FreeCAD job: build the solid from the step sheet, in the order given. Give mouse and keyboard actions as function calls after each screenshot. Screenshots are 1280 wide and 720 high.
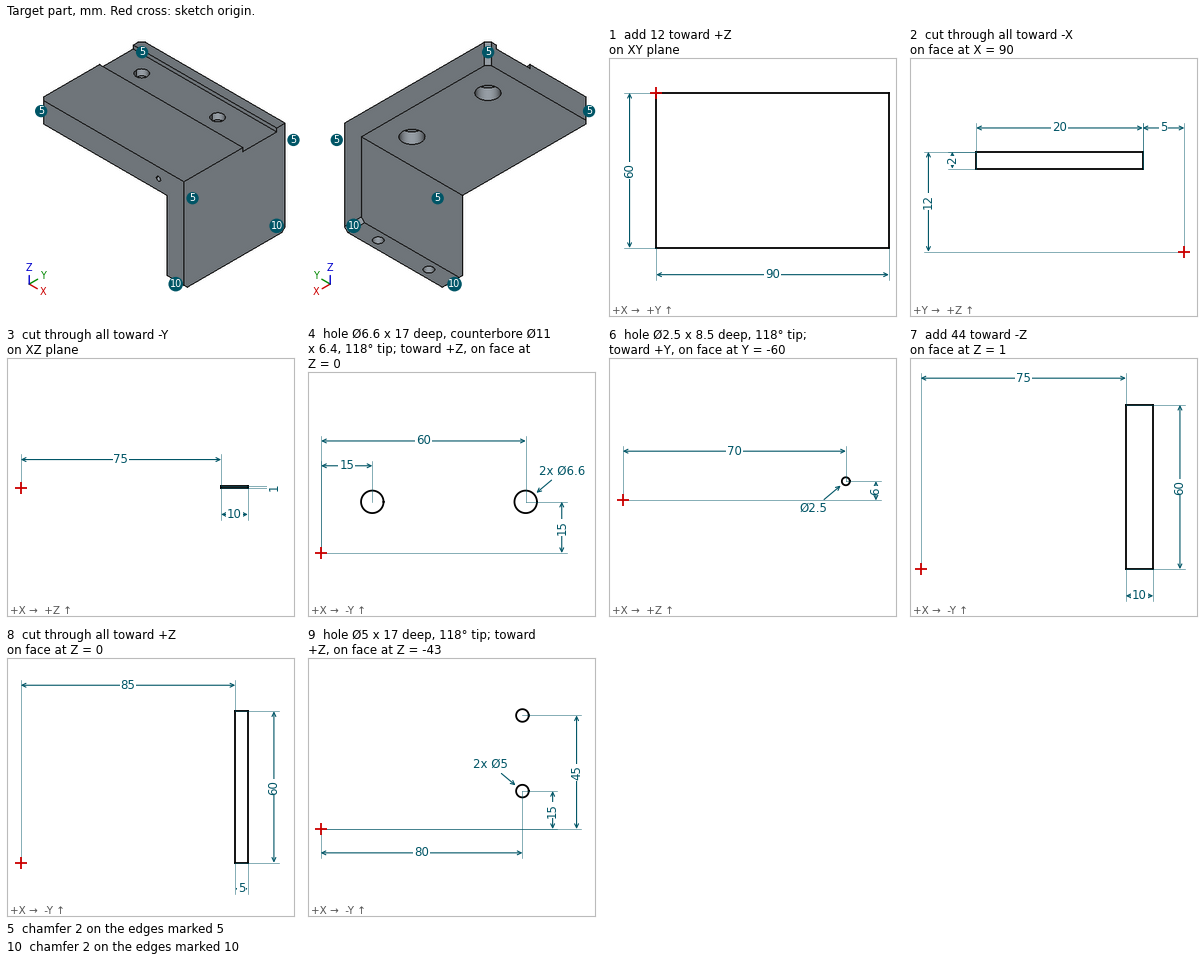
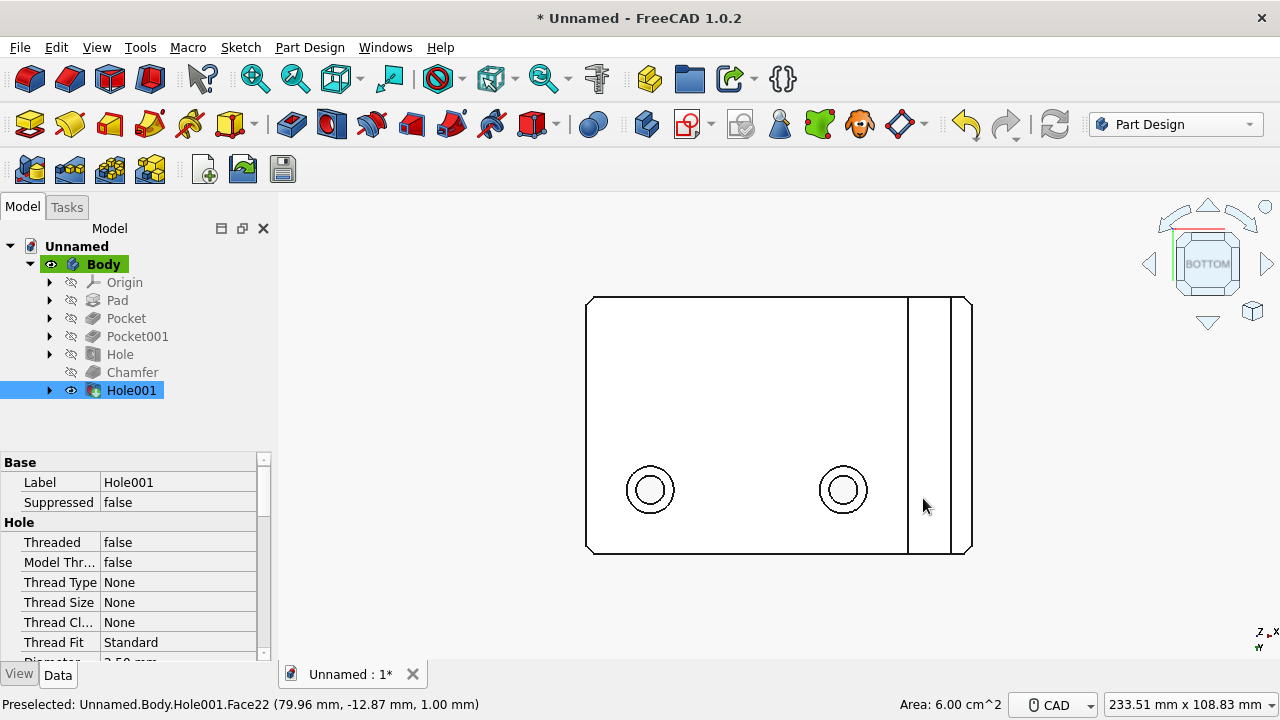
click(688, 124)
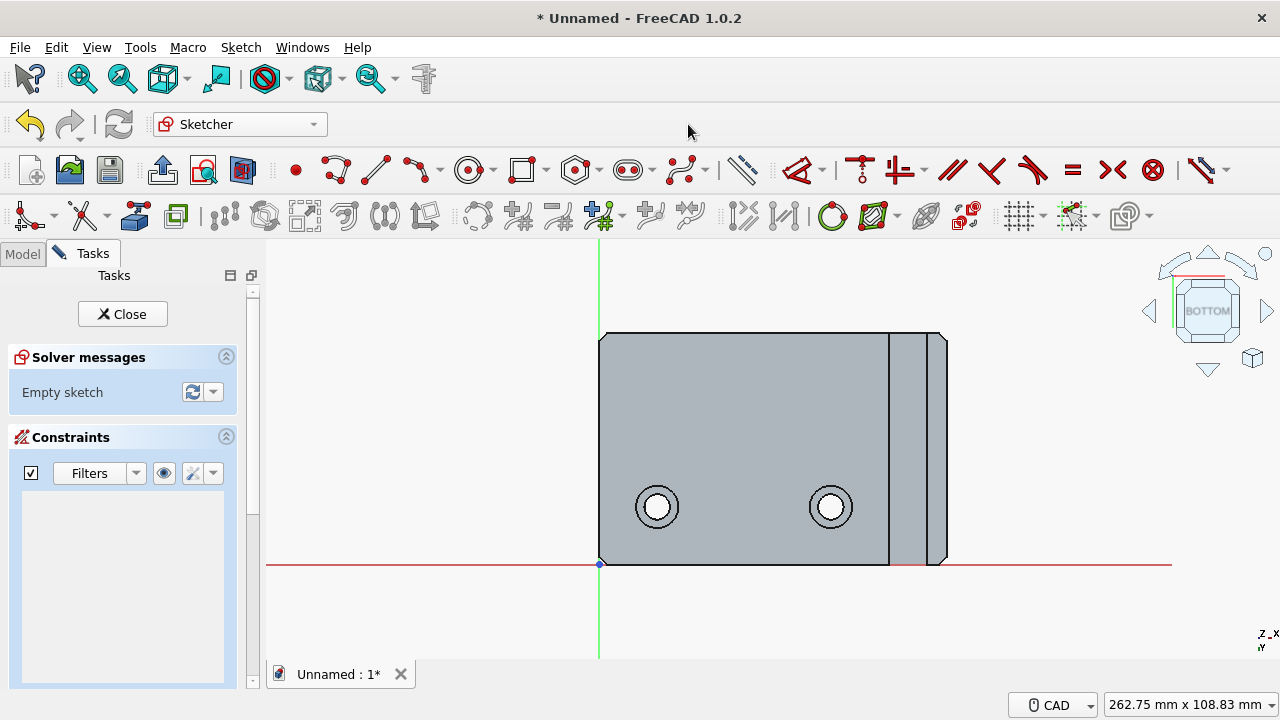
key(q)
key(s)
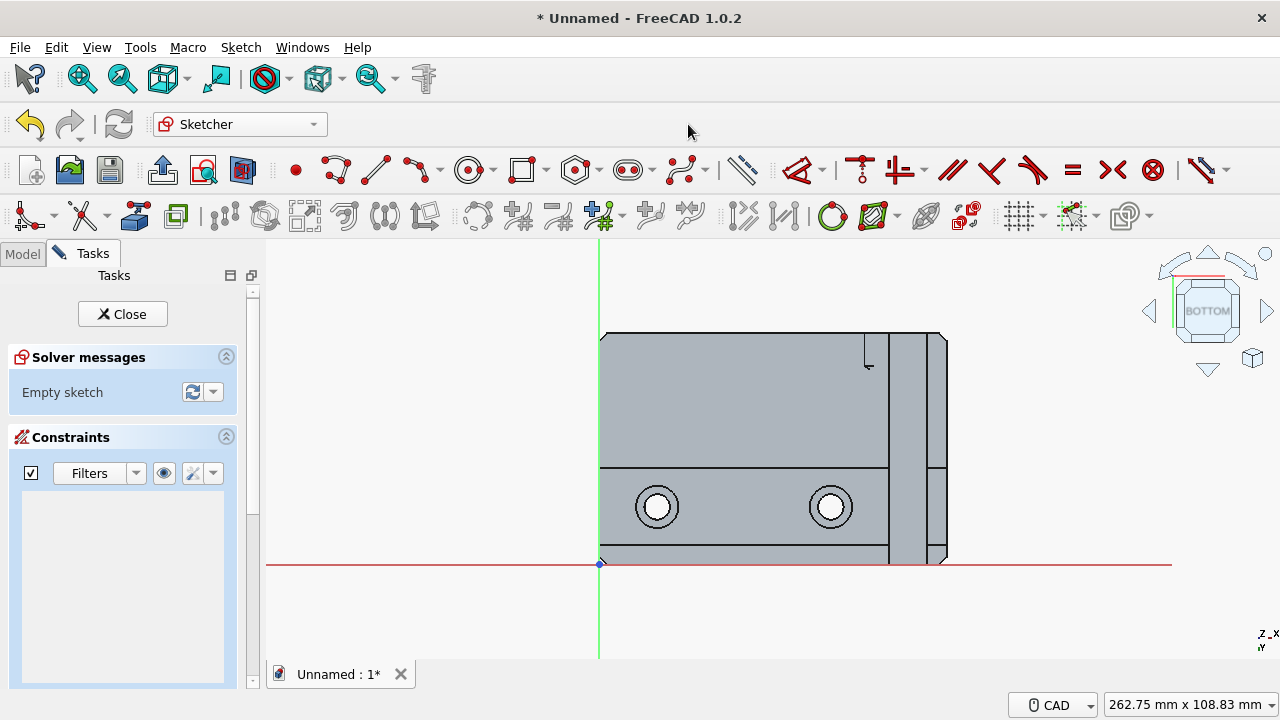
click(522, 170)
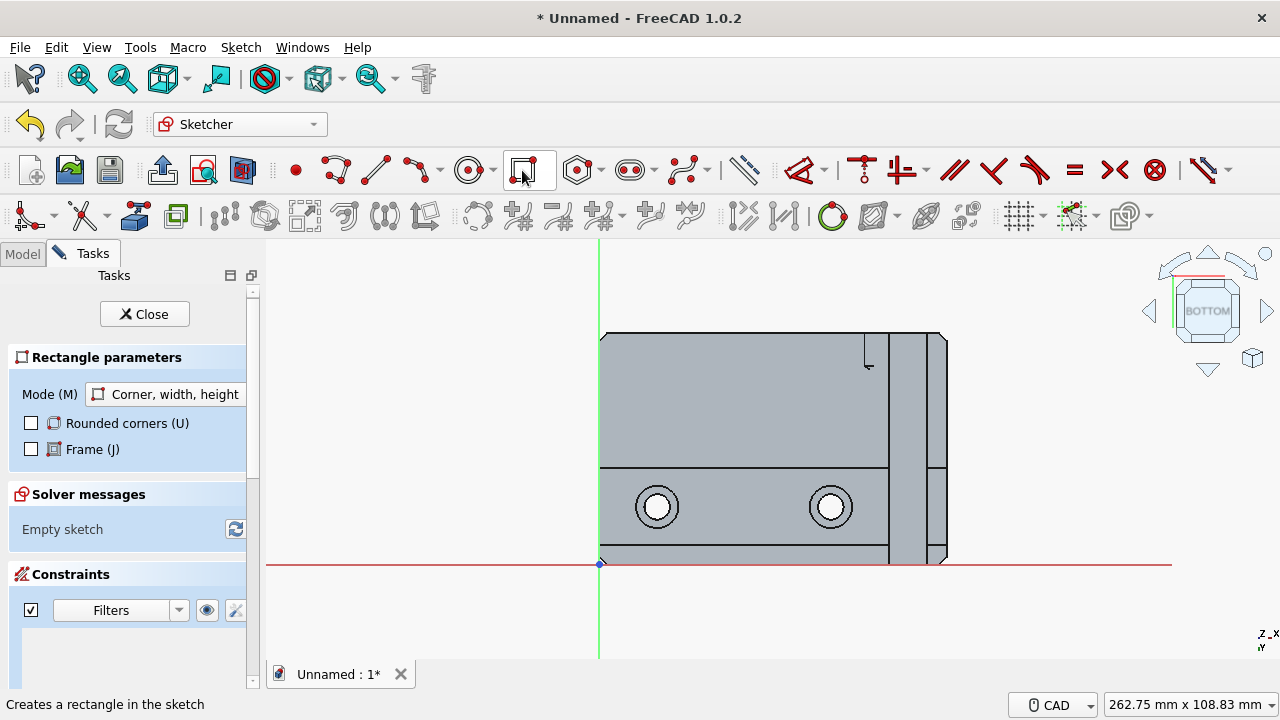
click(889, 333)
click(927, 565)
key(Escape)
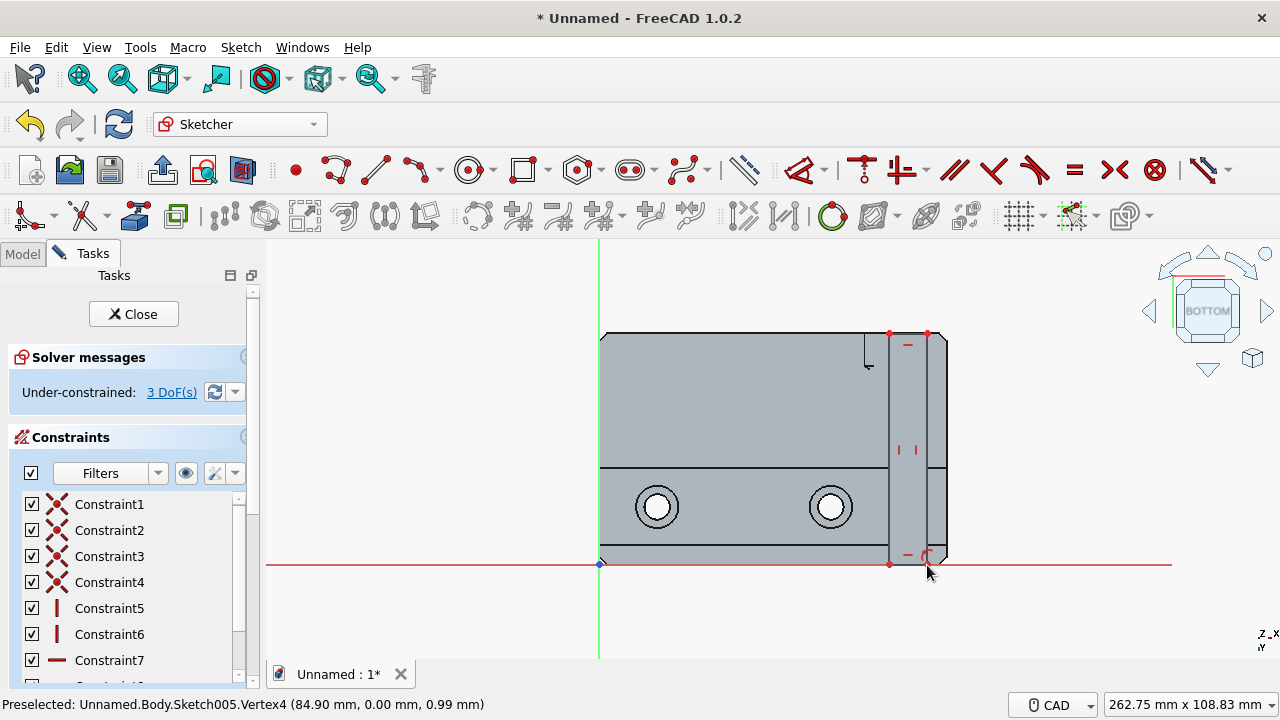
key(d)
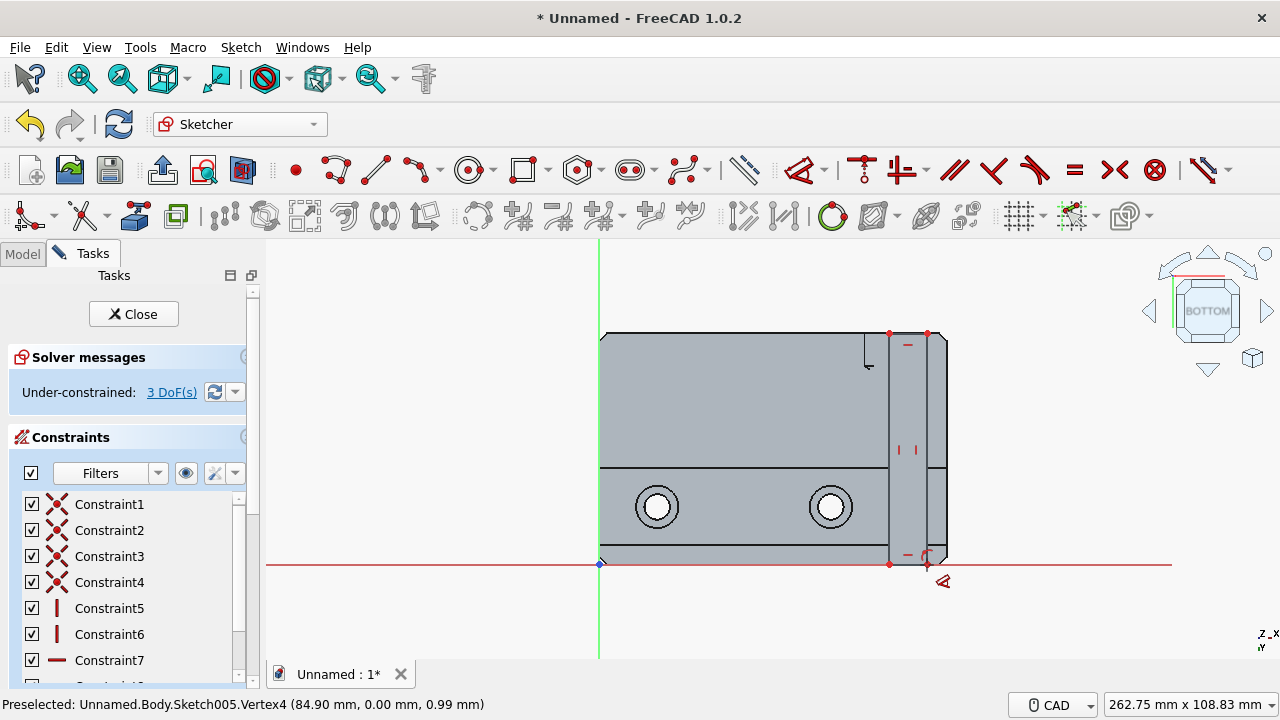
click(889, 403)
click(855, 449)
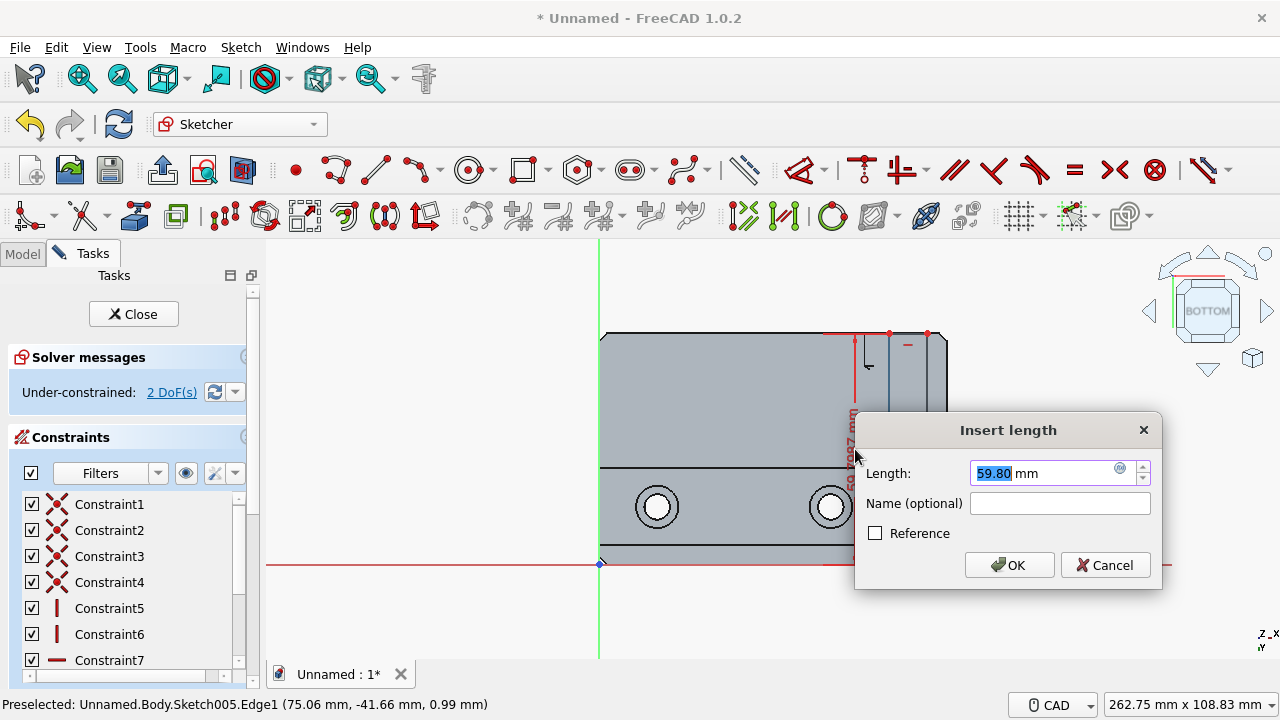
text(60)
key(Return)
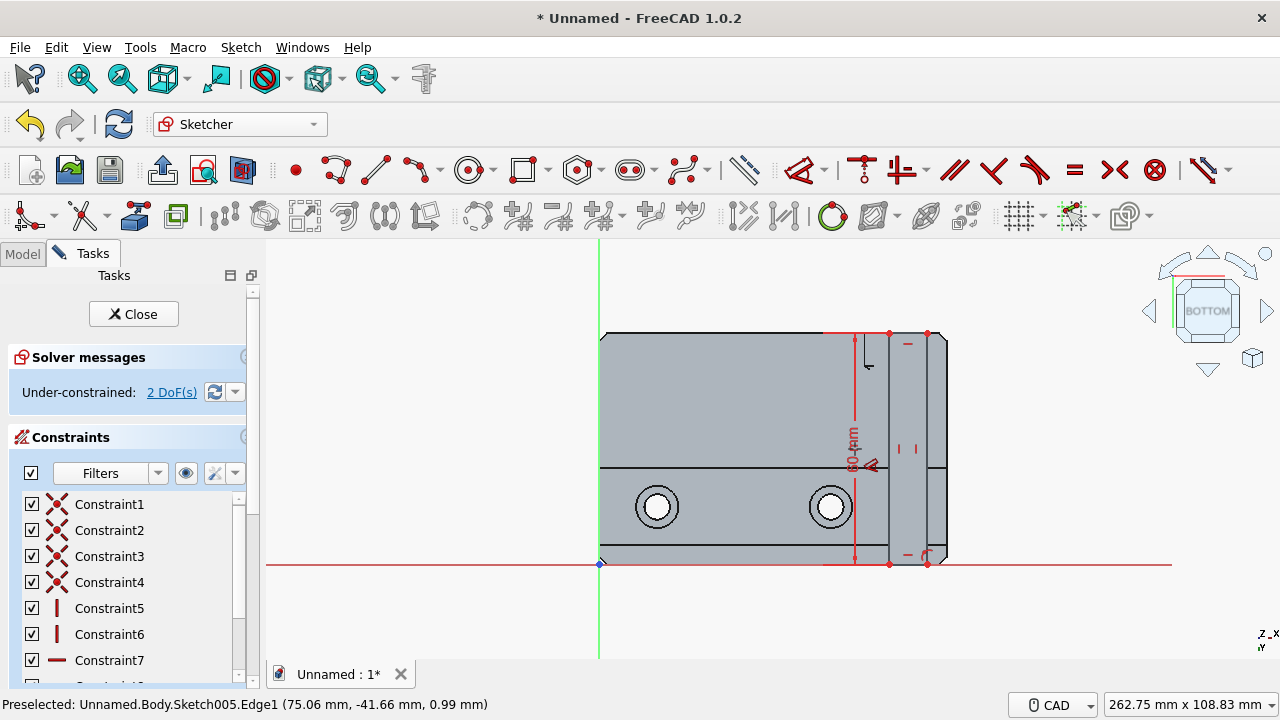
click(900, 565)
click(908, 599)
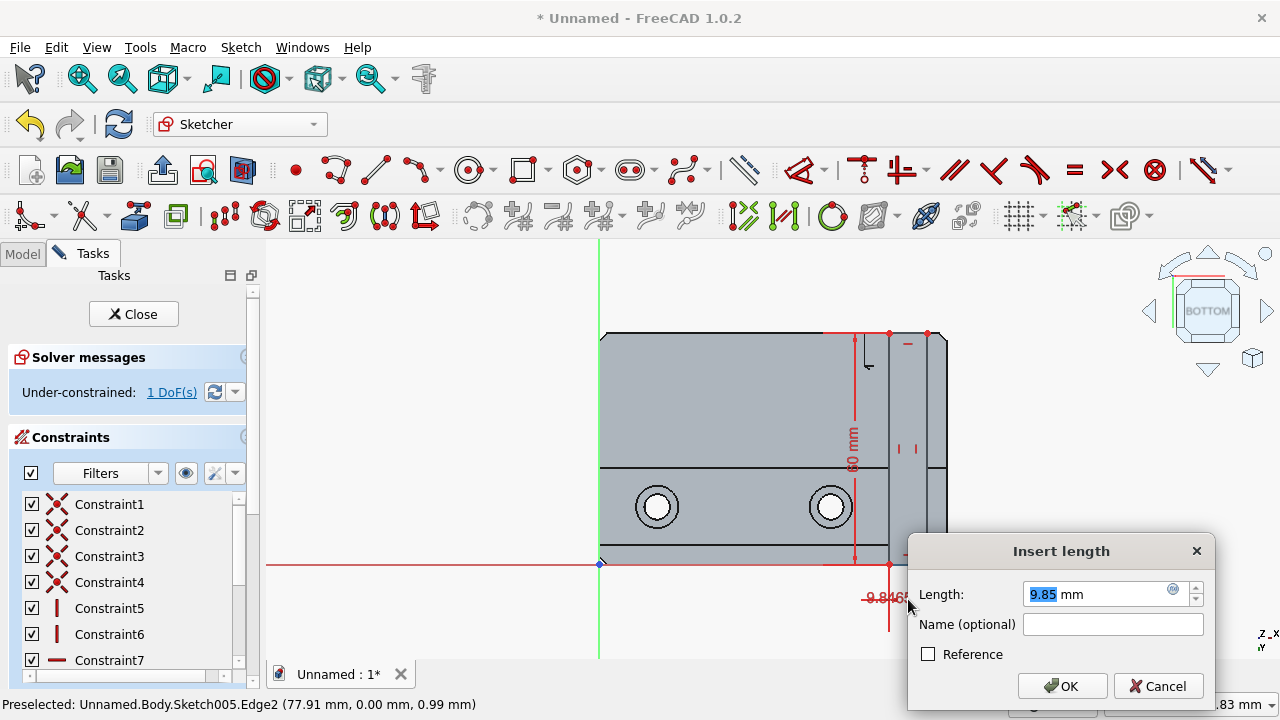
text(10)
key(Return)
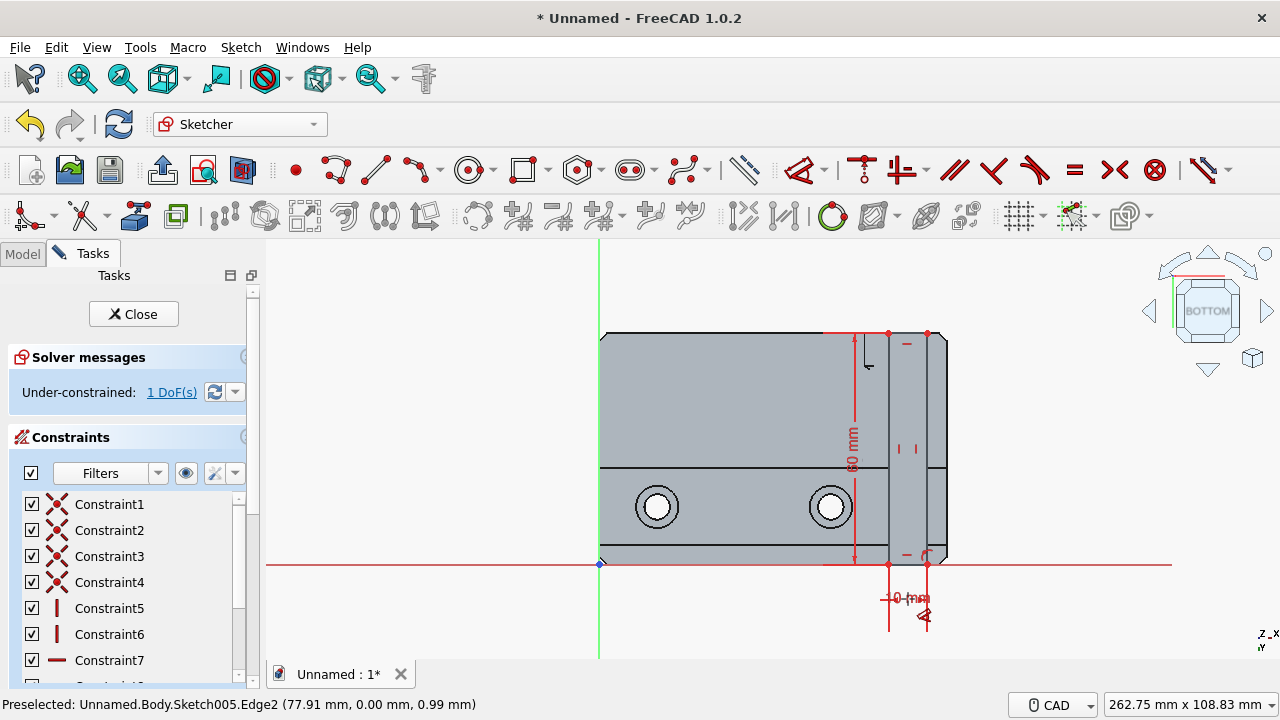
click(889, 333)
click(744, 599)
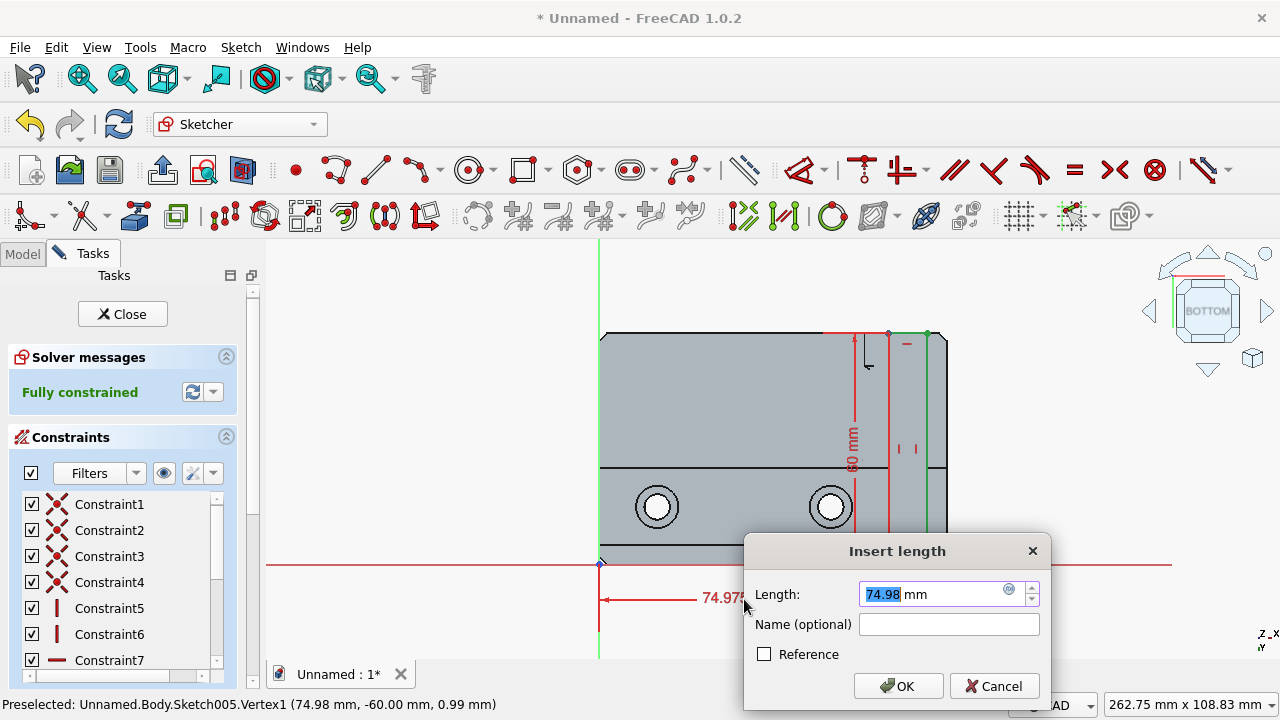
text(75)
key(Return)
key(Escape)